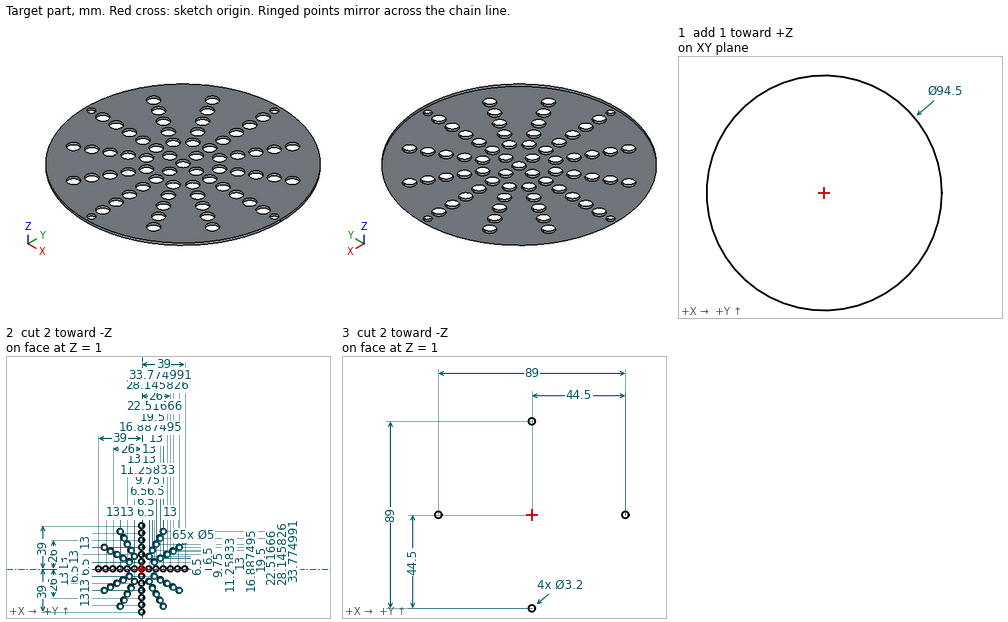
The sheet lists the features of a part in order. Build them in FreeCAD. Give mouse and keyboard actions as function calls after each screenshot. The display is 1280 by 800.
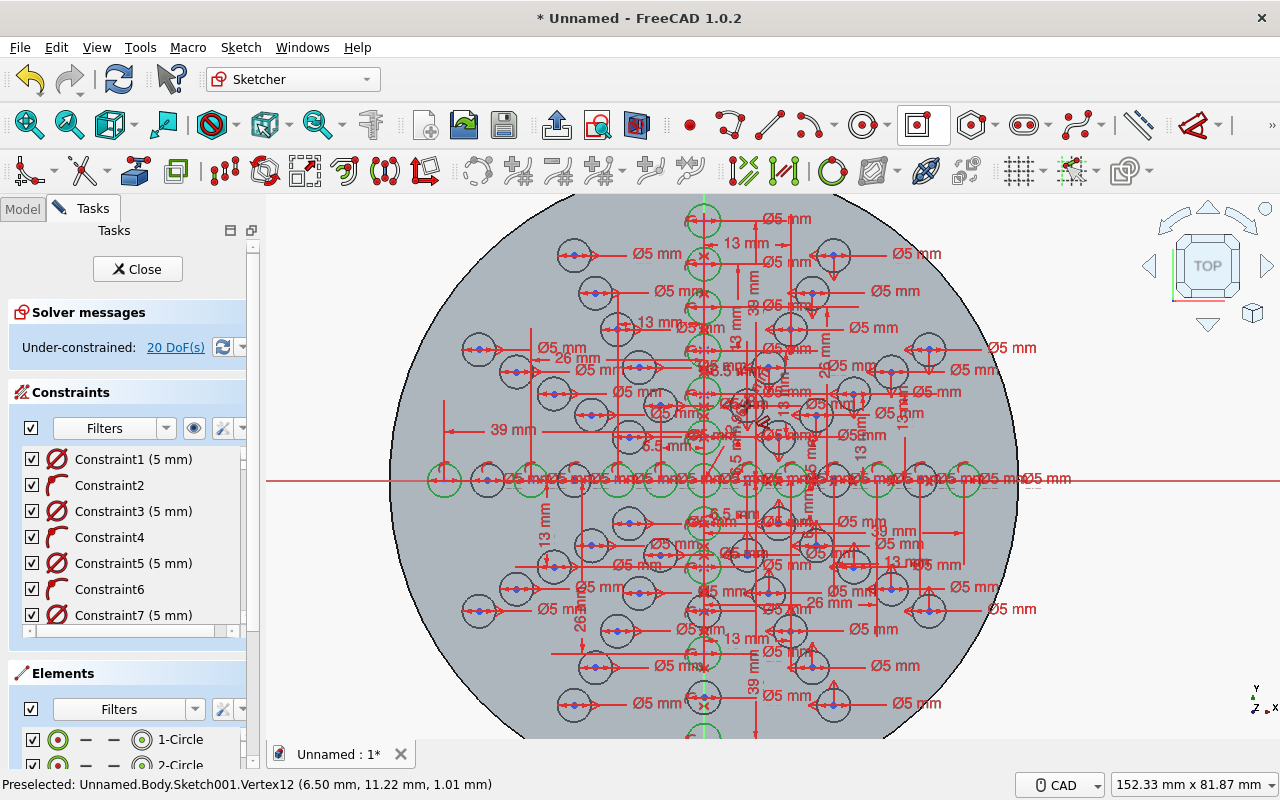
click(834, 481)
click(821, 324)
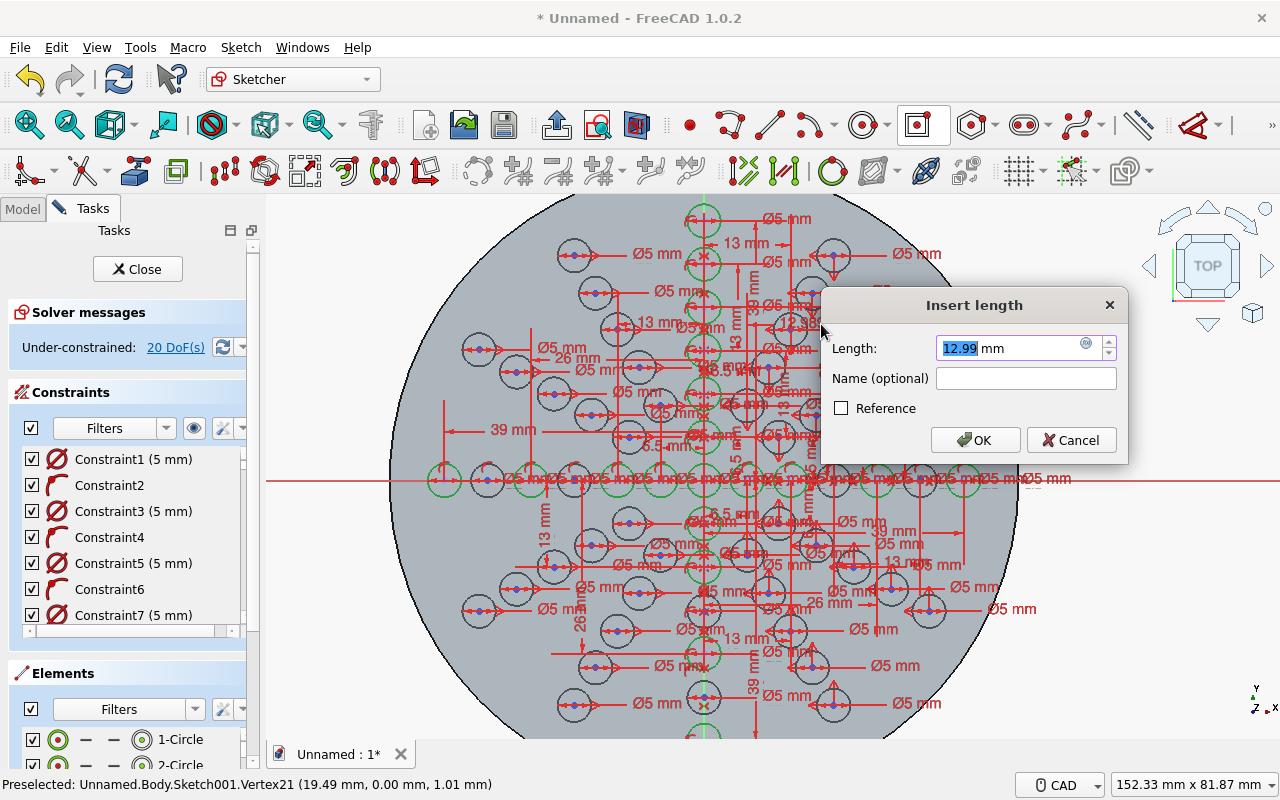
text(13)
key(Return)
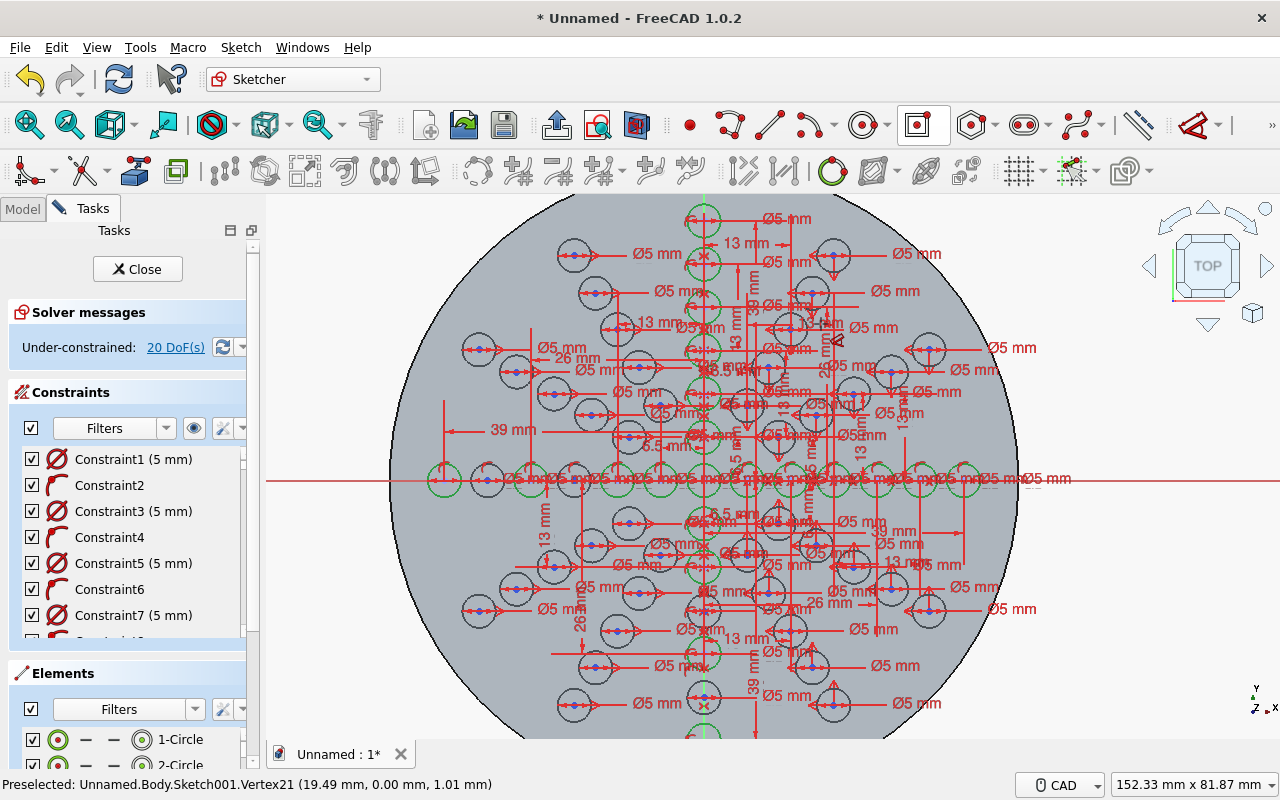
click(704, 698)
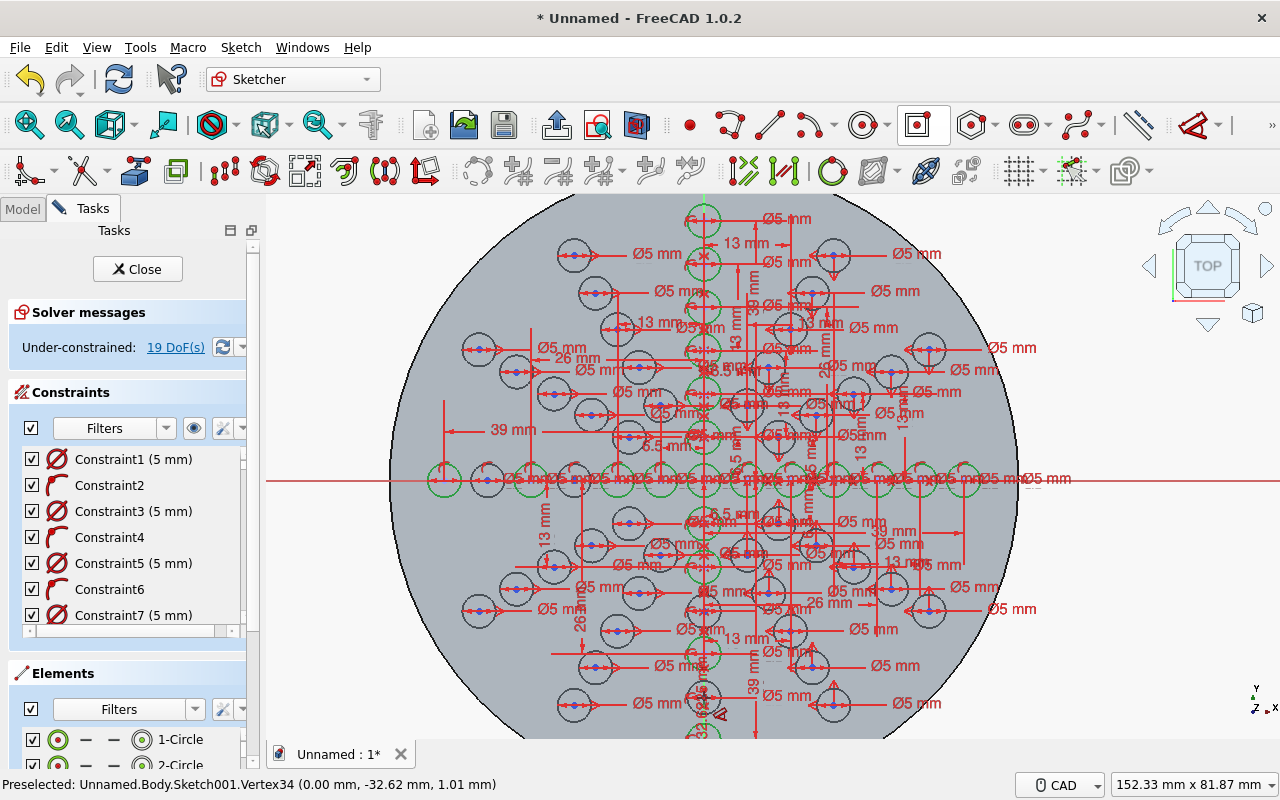
click(704, 611)
click(670, 654)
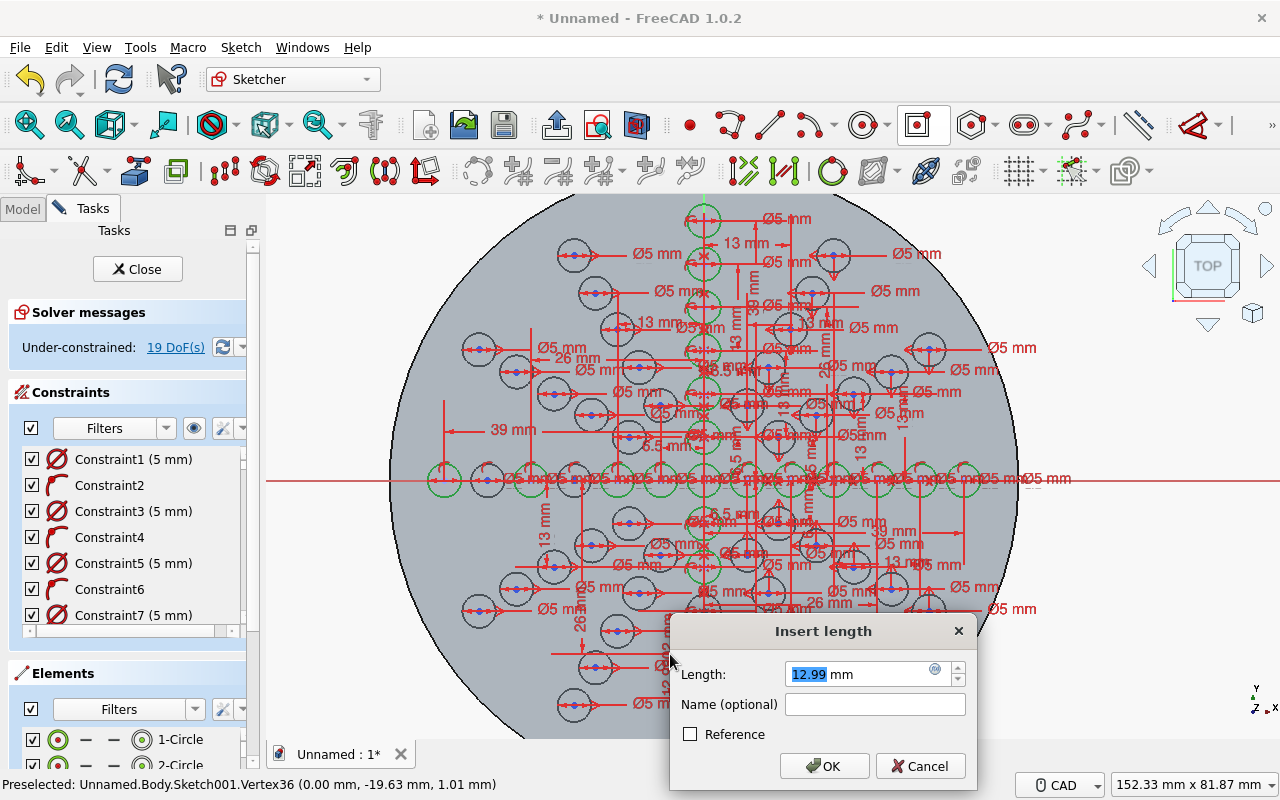
text(13)
key(Return)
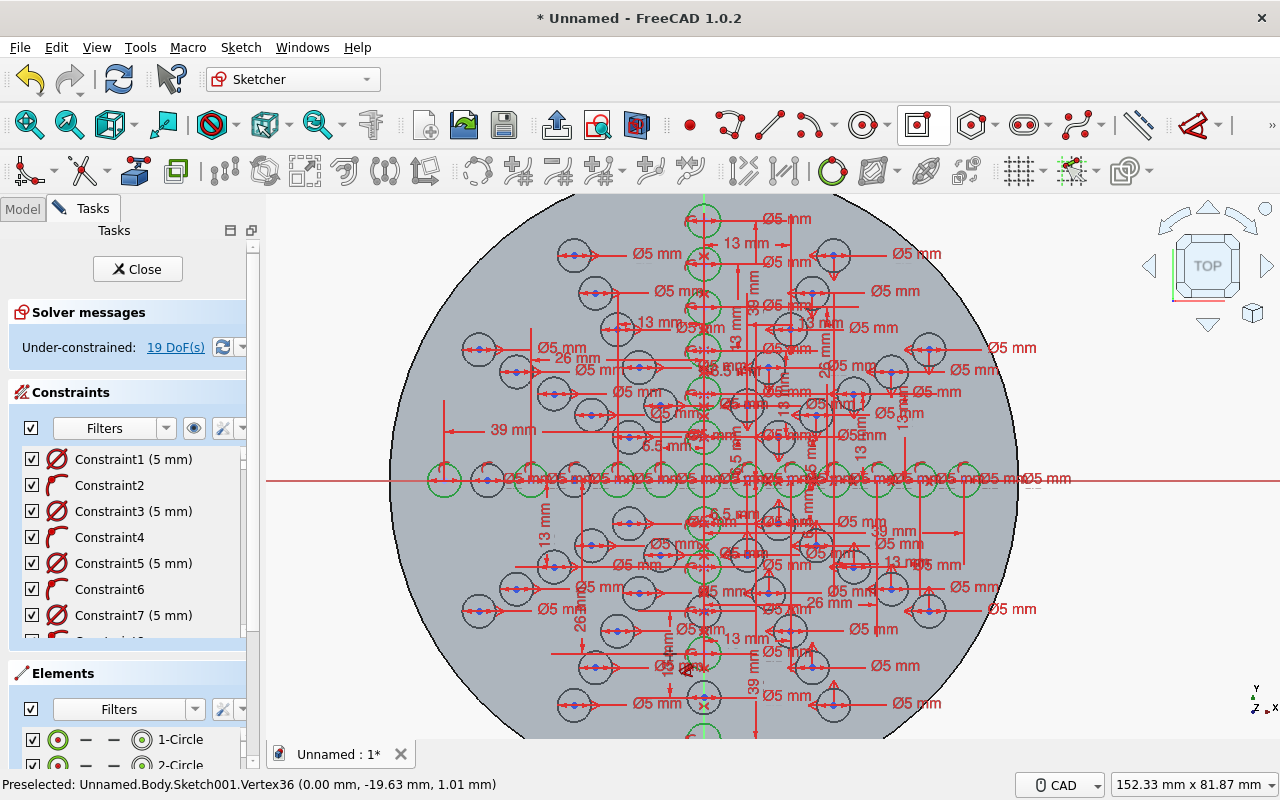
click(779, 524)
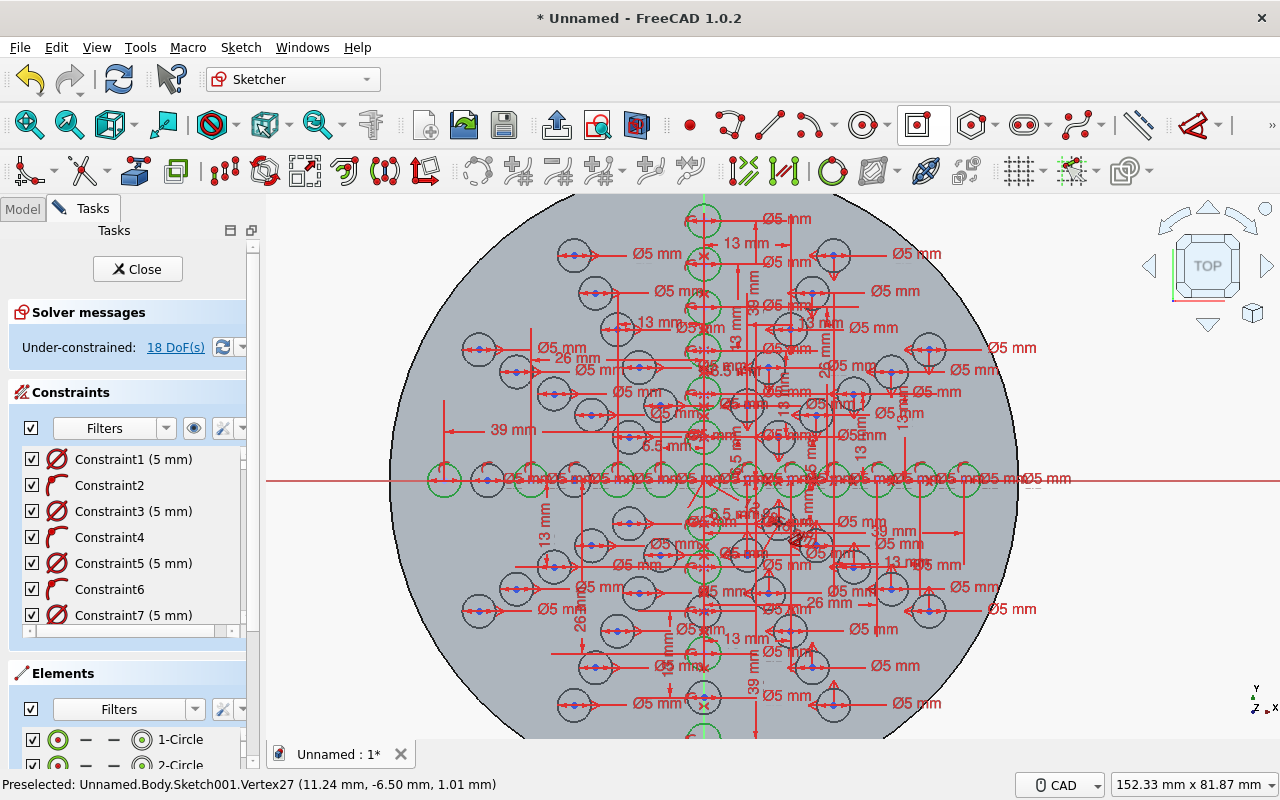
click(704, 611)
click(670, 588)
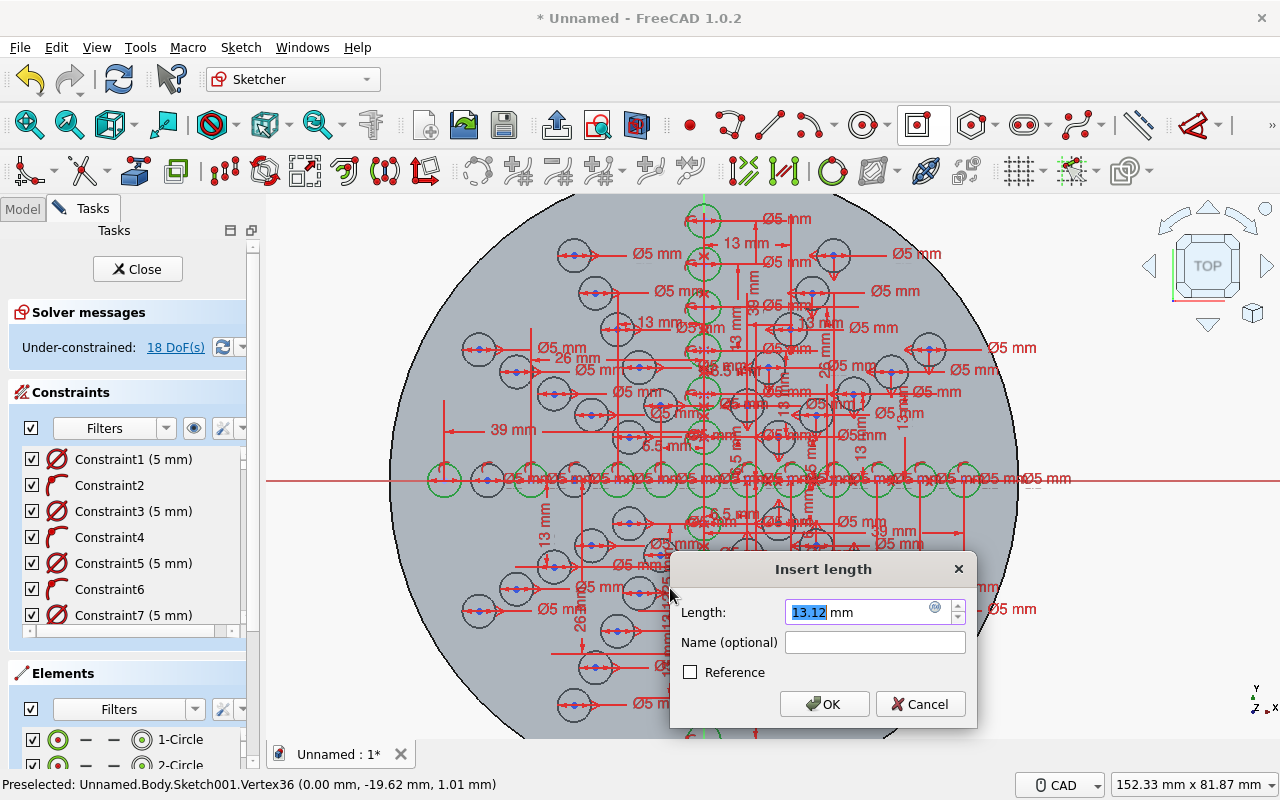
text(13)
key(Return)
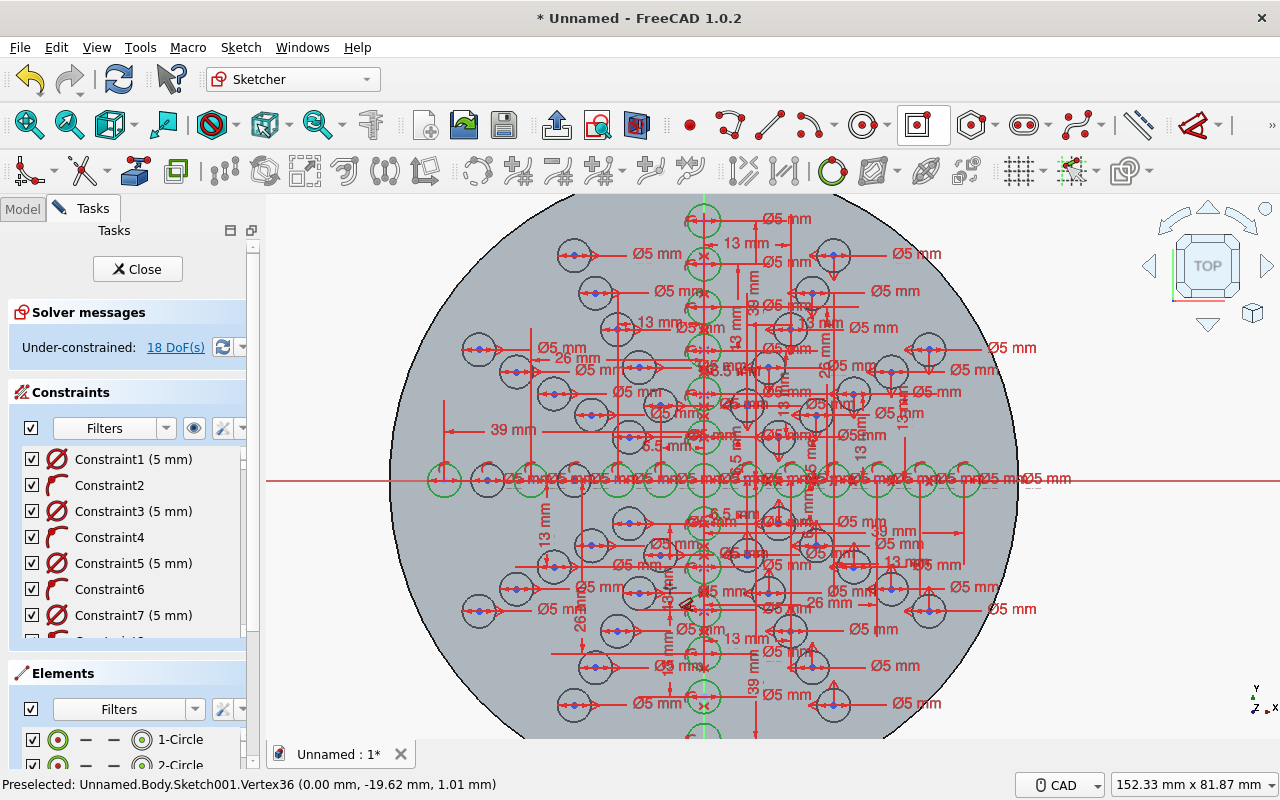
click(488, 481)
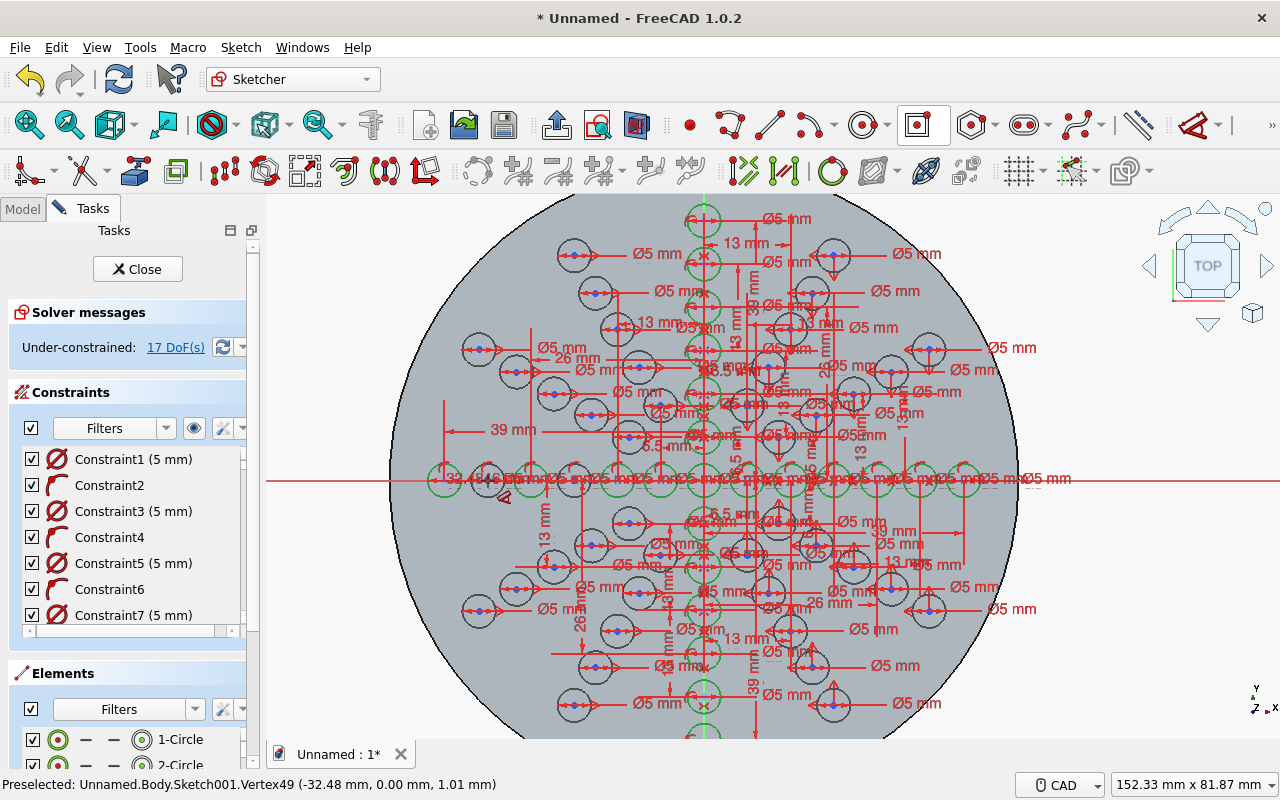
click(574, 481)
click(501, 563)